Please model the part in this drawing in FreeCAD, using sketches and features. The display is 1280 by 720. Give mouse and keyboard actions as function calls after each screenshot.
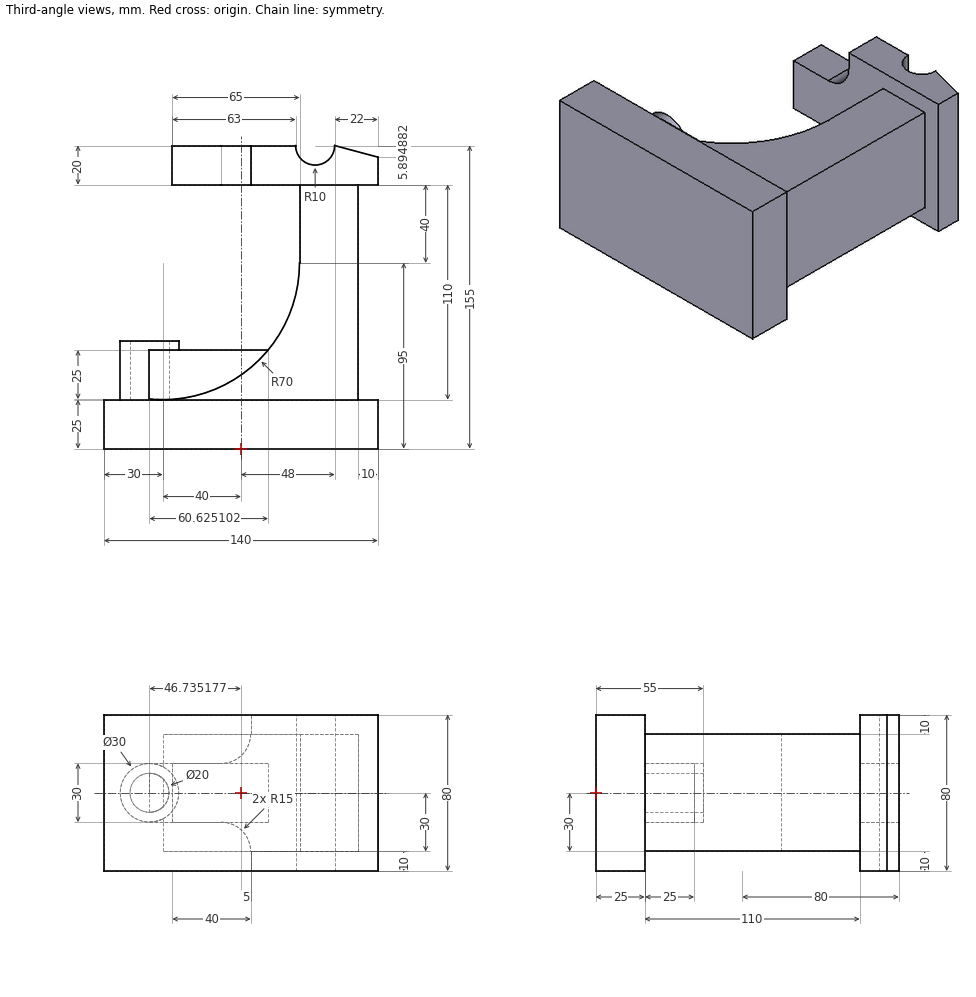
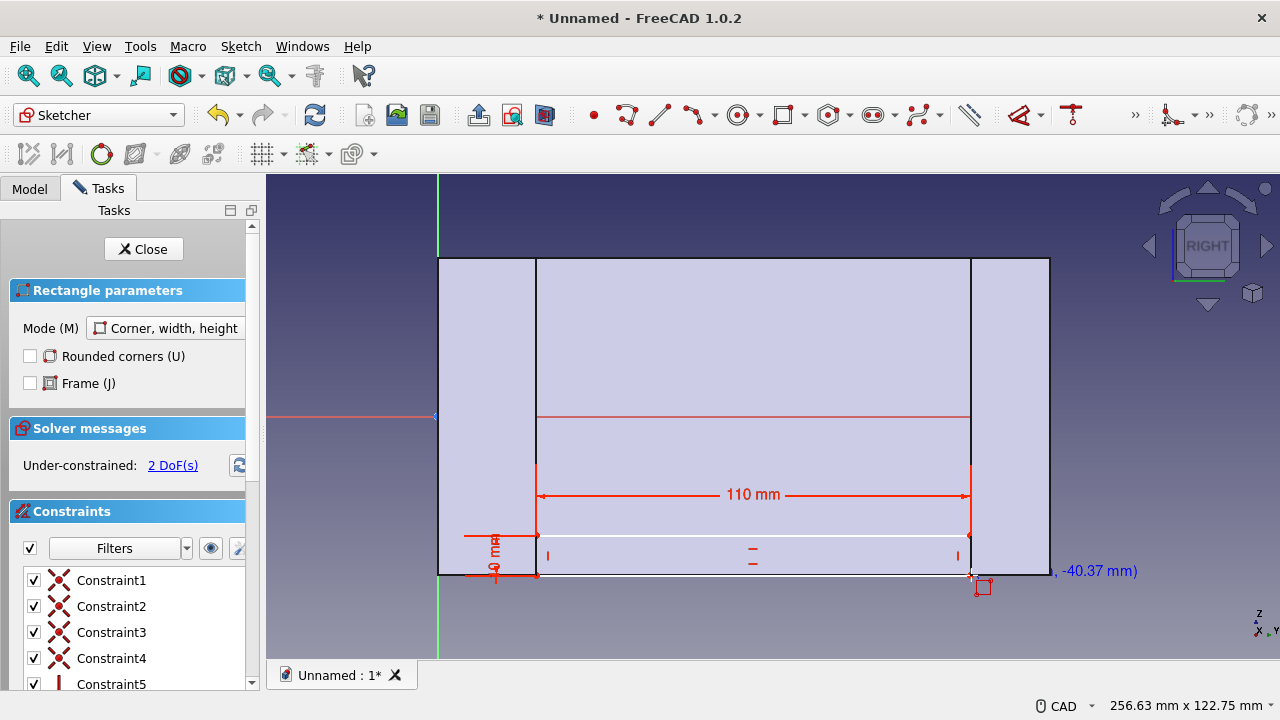
click(536, 258)
move(971, 298)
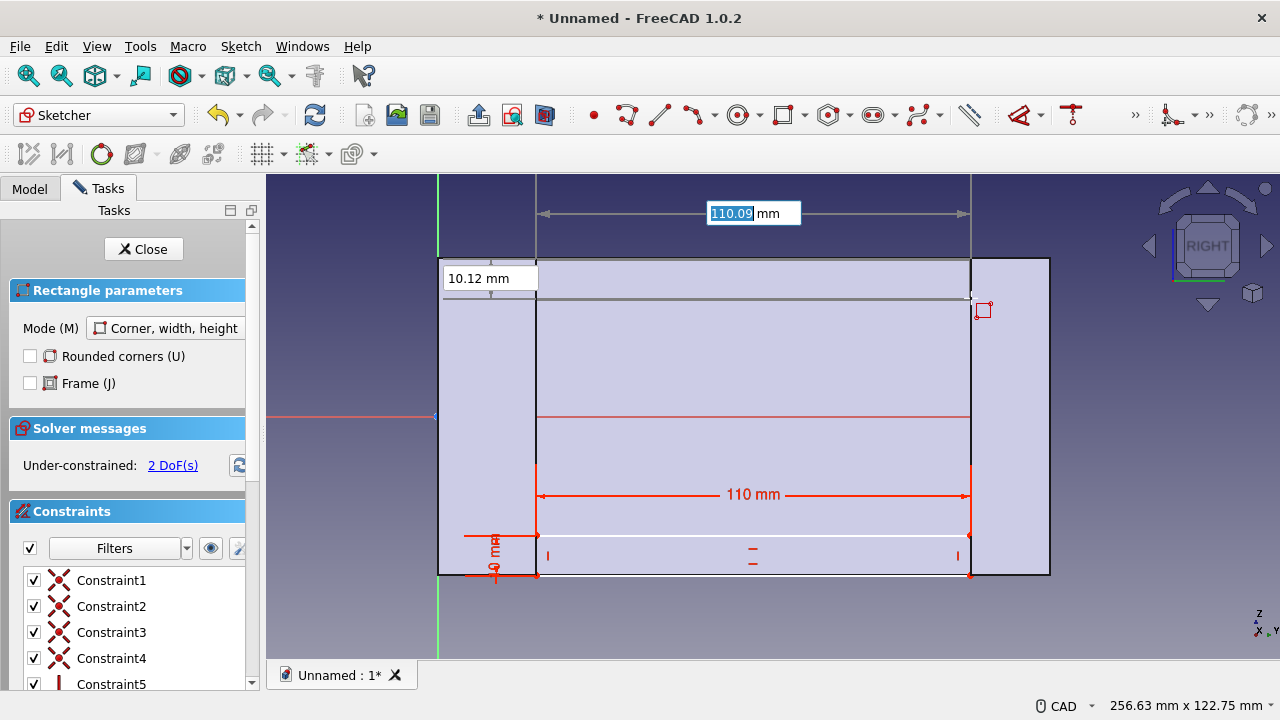
text(110)
key(Tab)
text(10)
key(Return)
key(Escape)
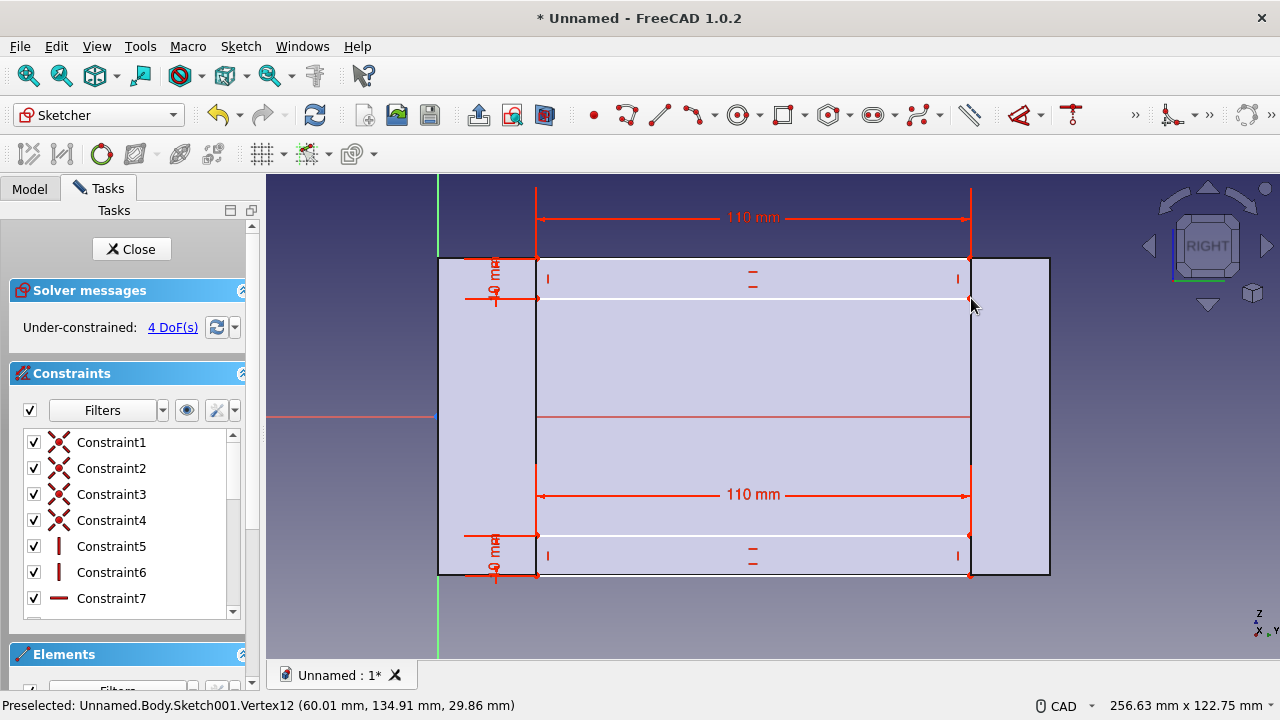
click(536, 576)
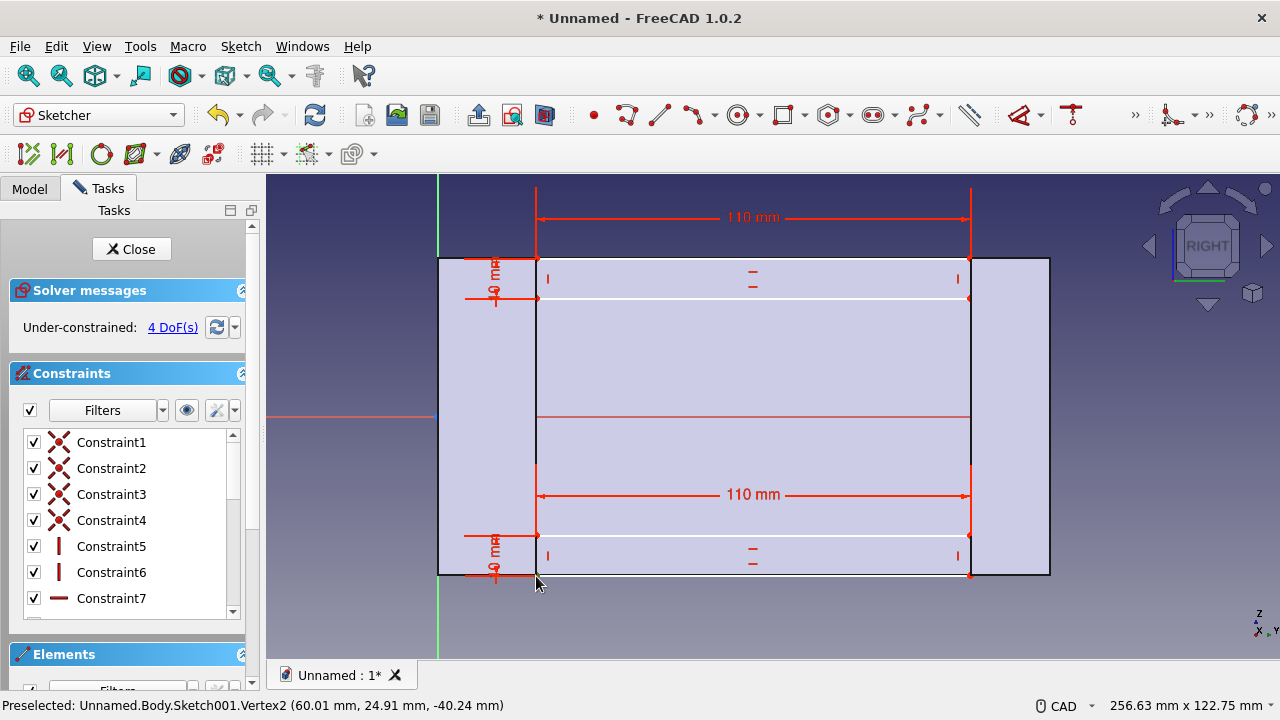
click(536, 259)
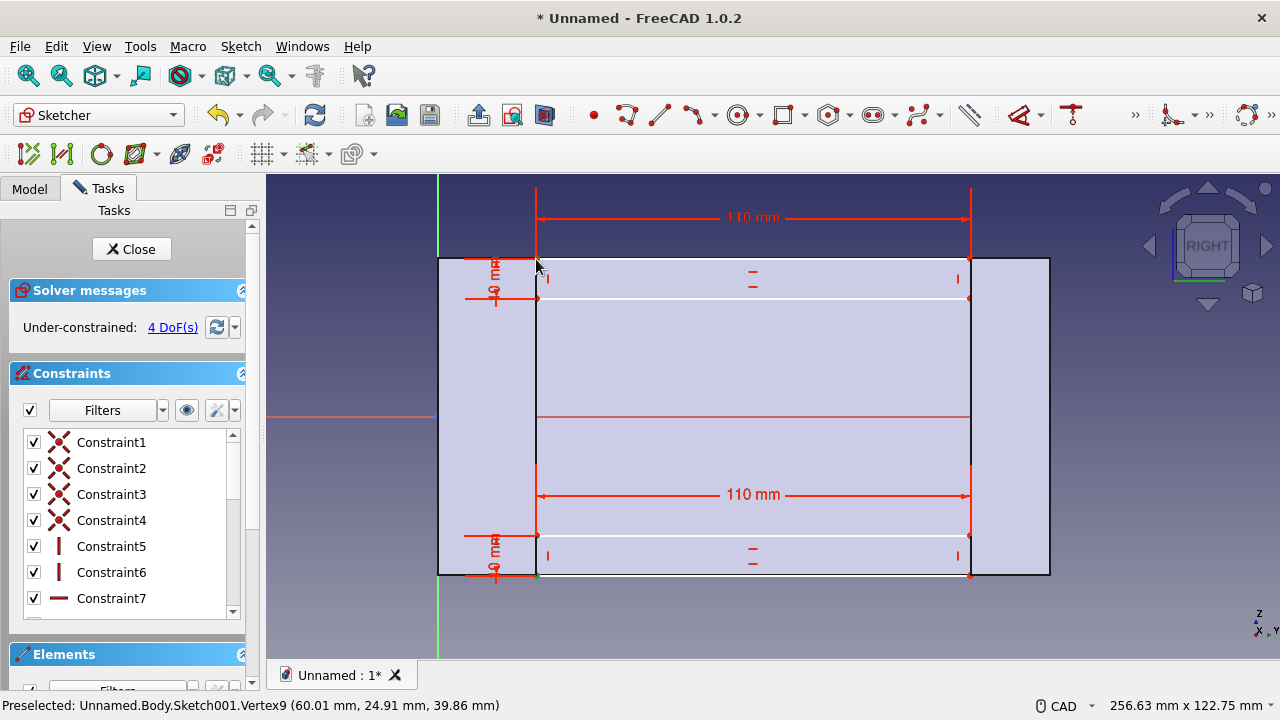
click(353, 416)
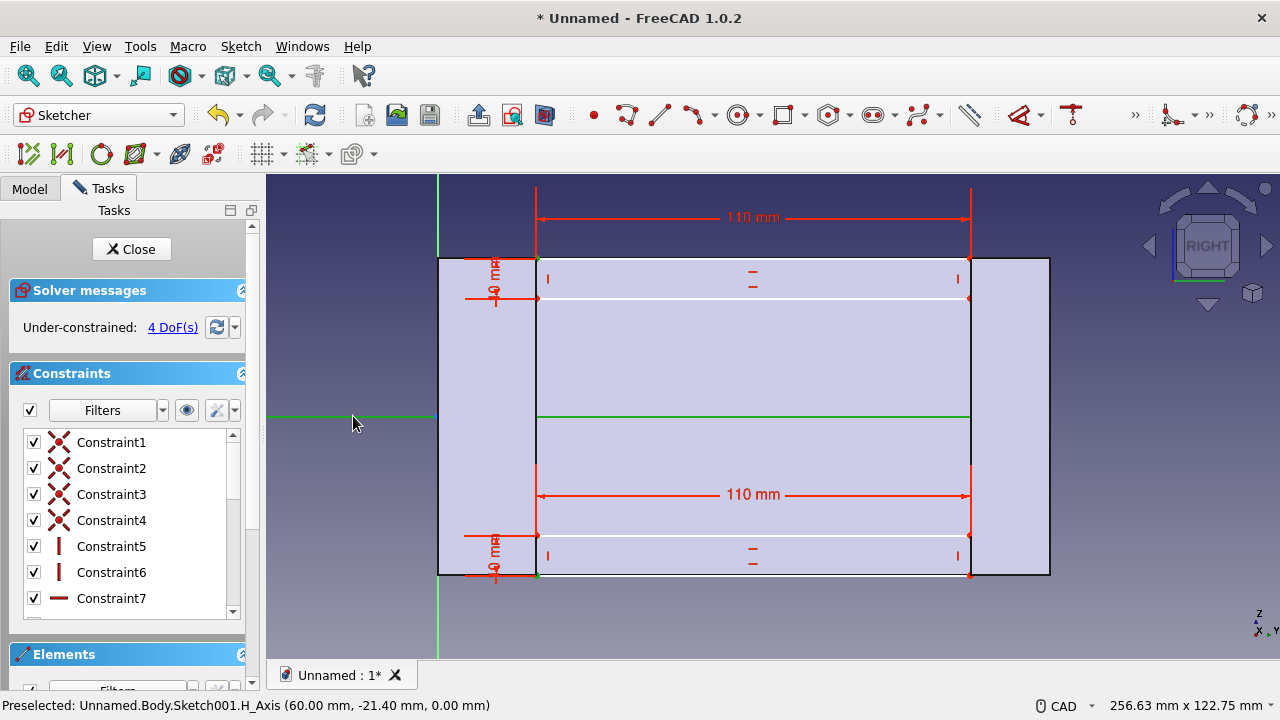
key(s)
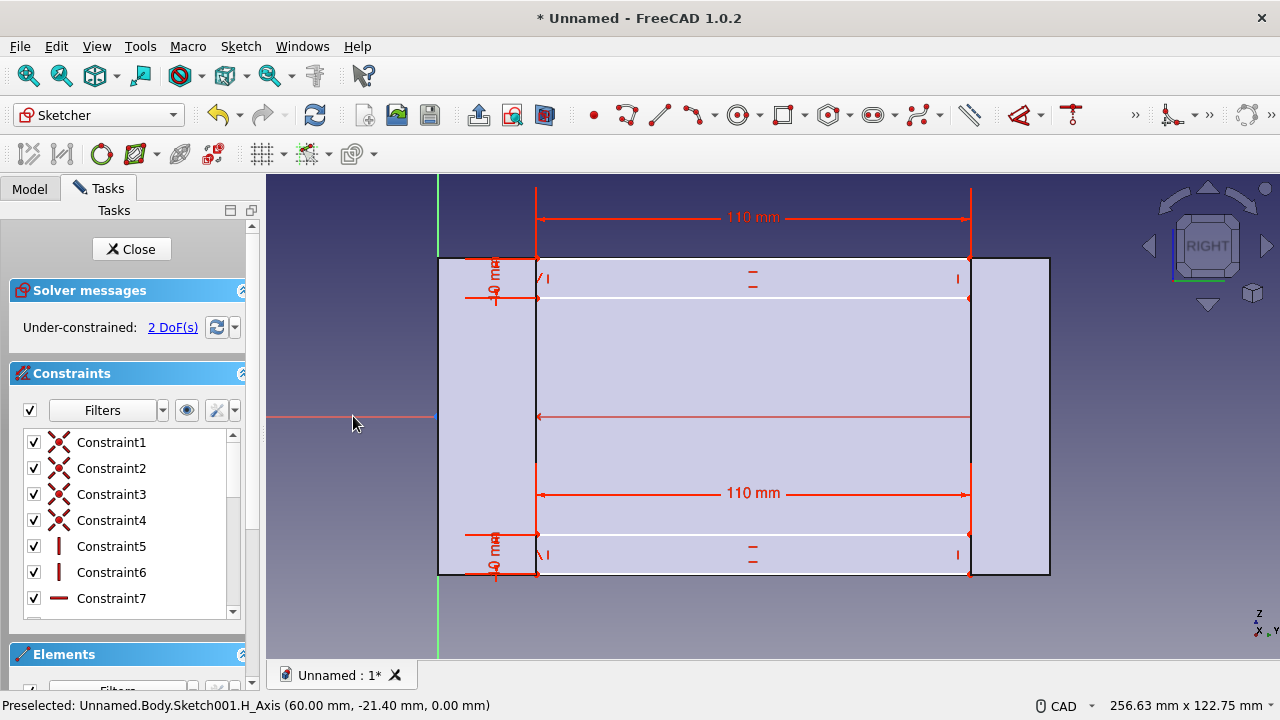
click(1018, 116)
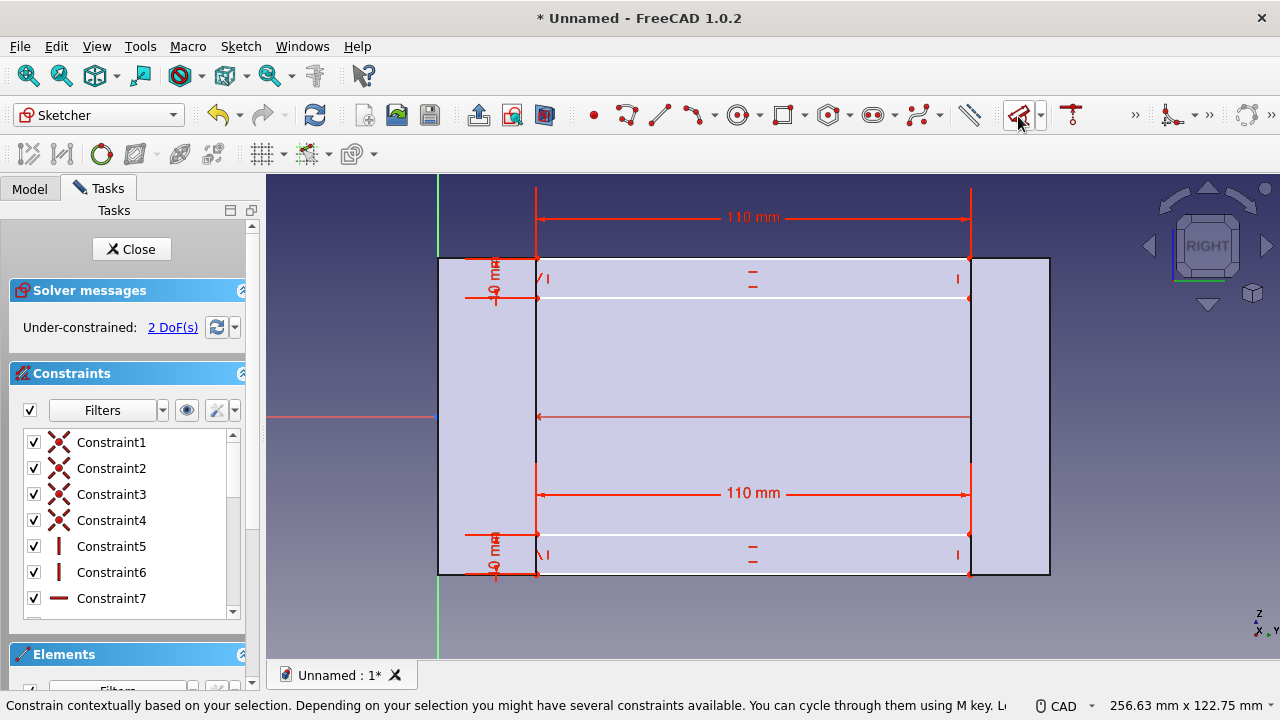
click(536, 535)
click(487, 569)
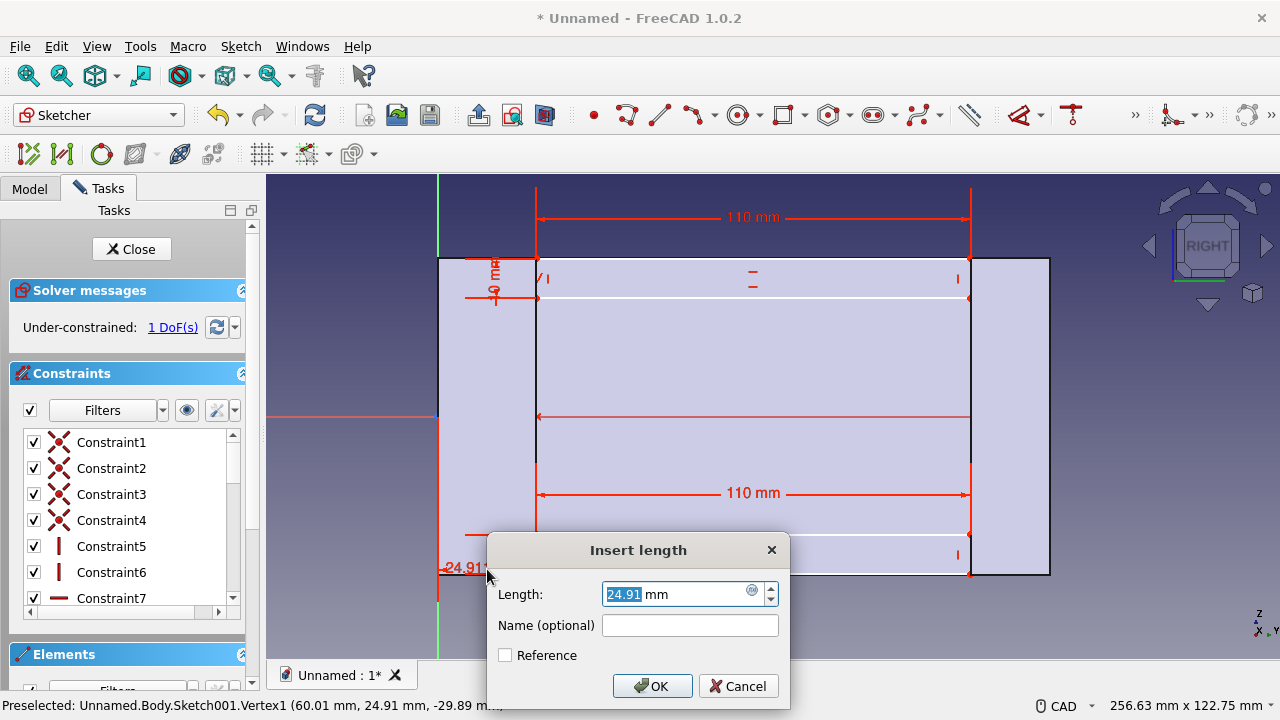
text(25)
key(Return)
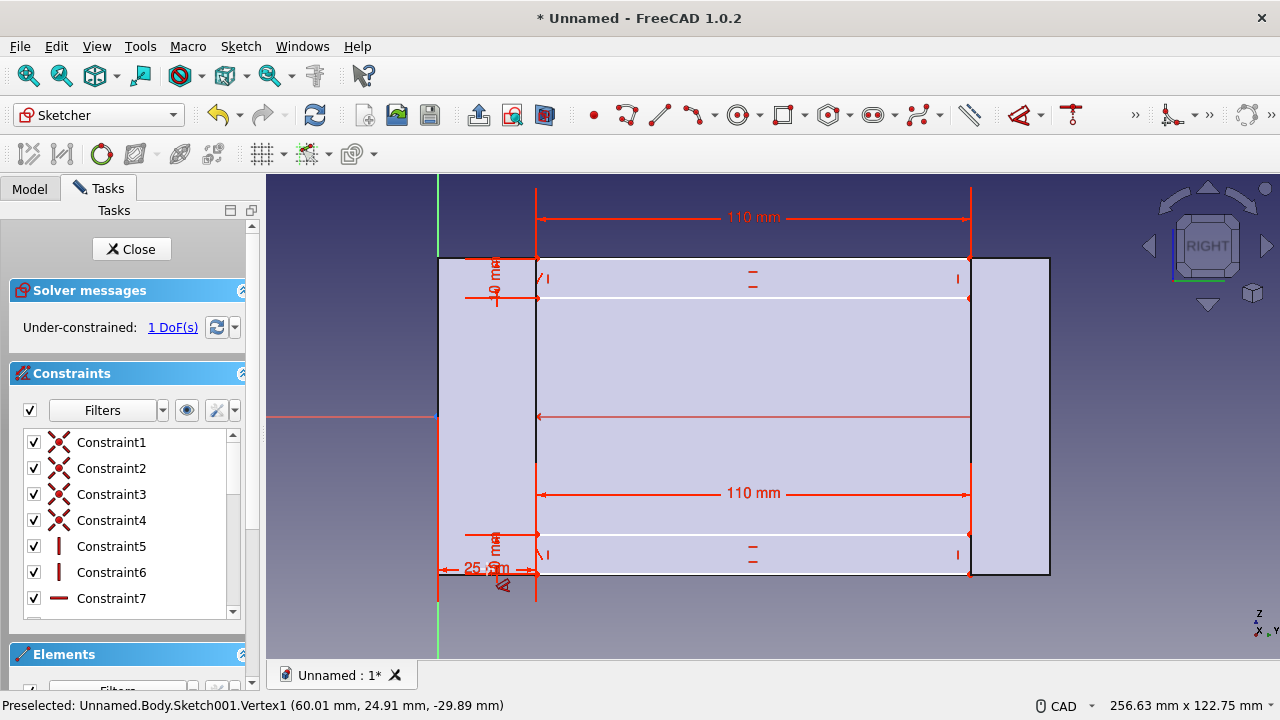
click(536, 535)
click(404, 476)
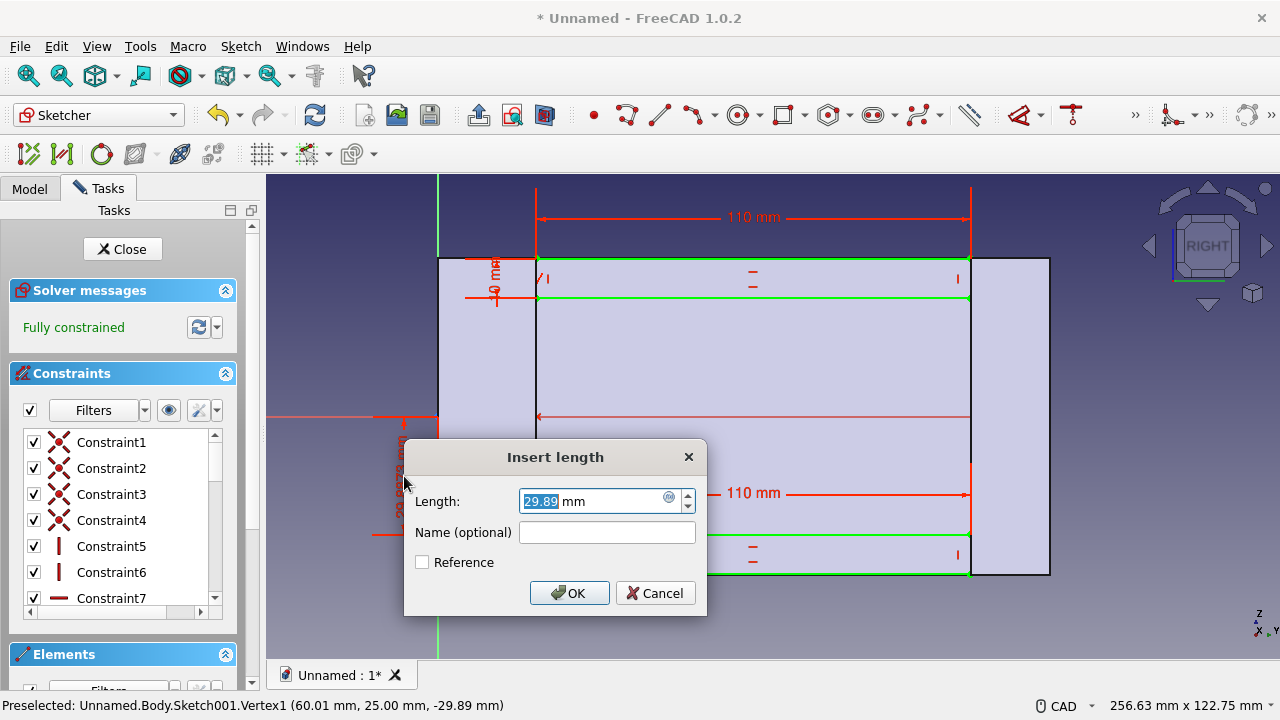
text(30)
key(Return)
key(Escape)